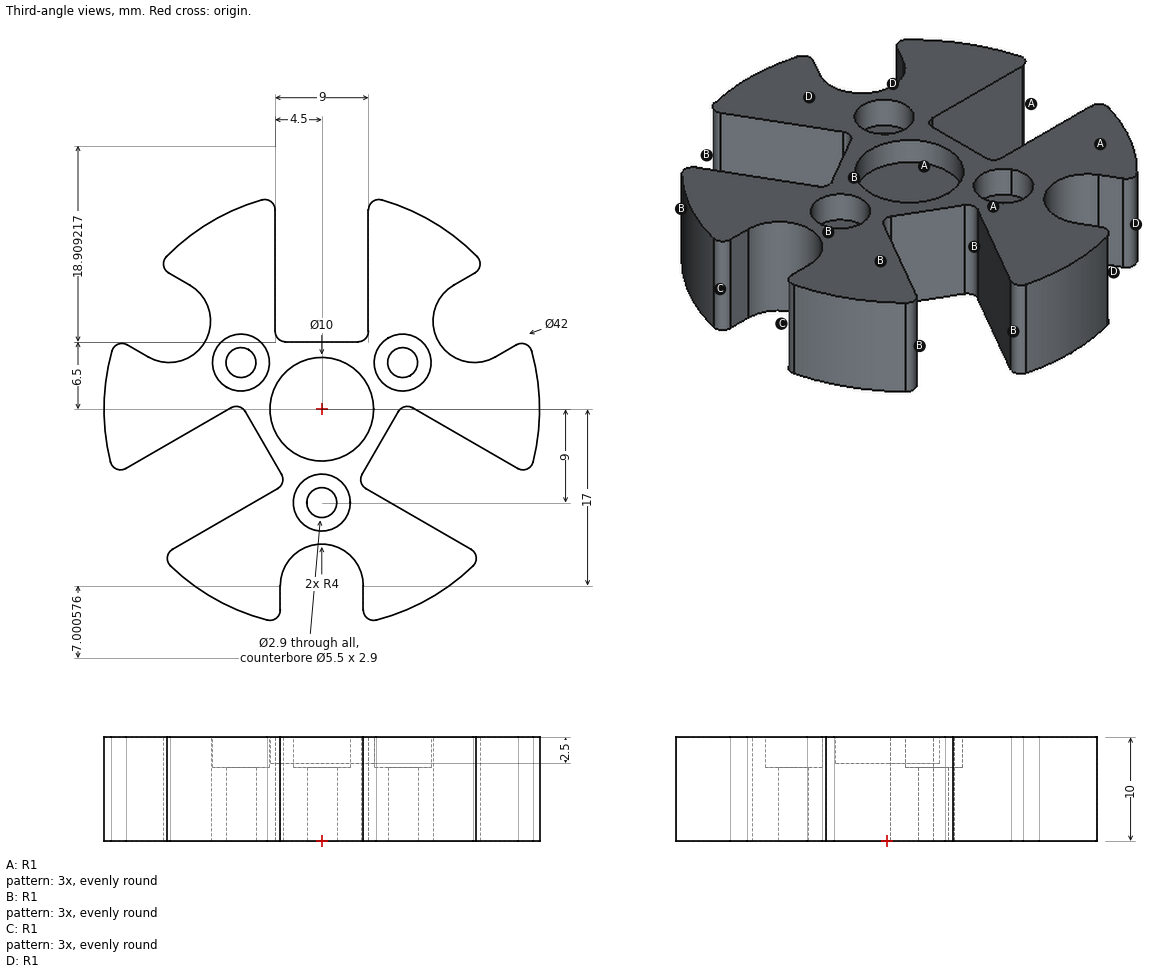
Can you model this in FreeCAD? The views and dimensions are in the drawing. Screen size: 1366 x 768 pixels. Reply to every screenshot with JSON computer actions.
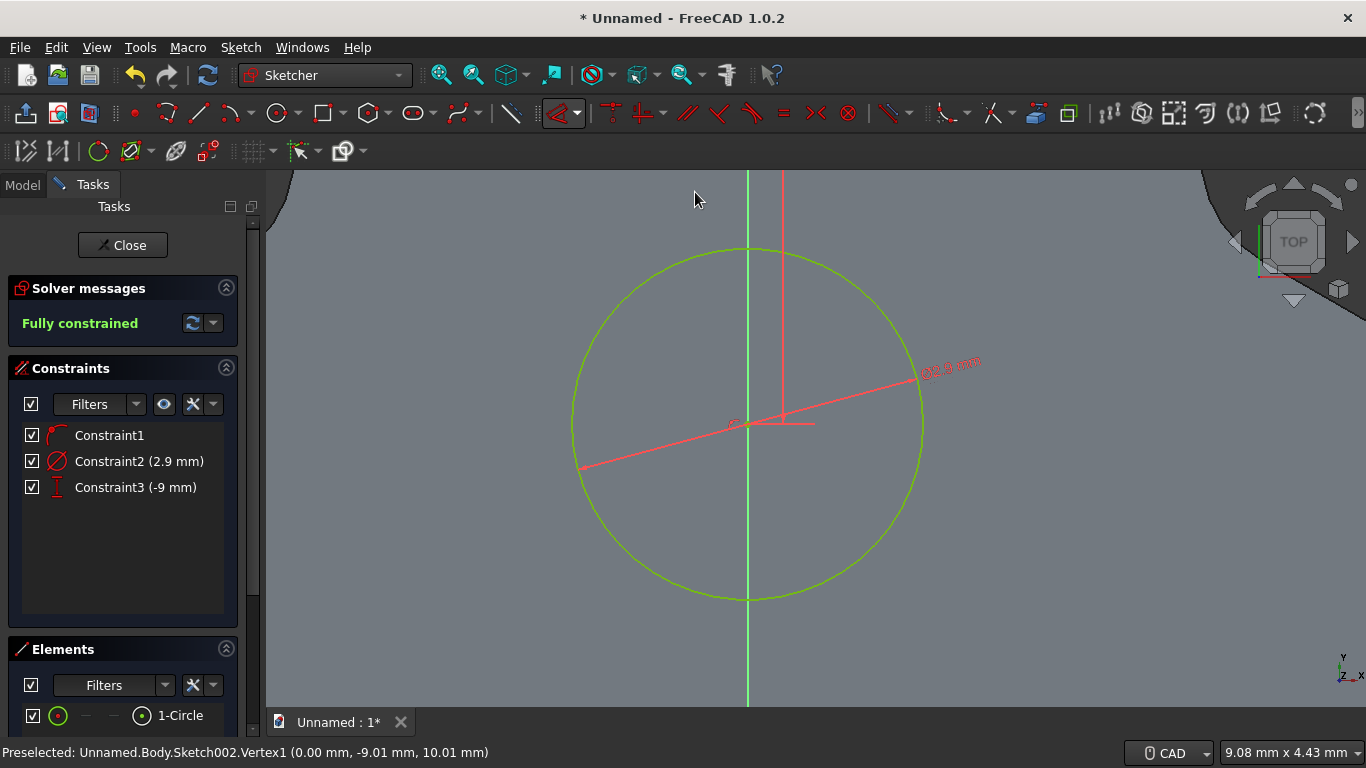
{"action": "left_click", "coordinate": [123, 245]}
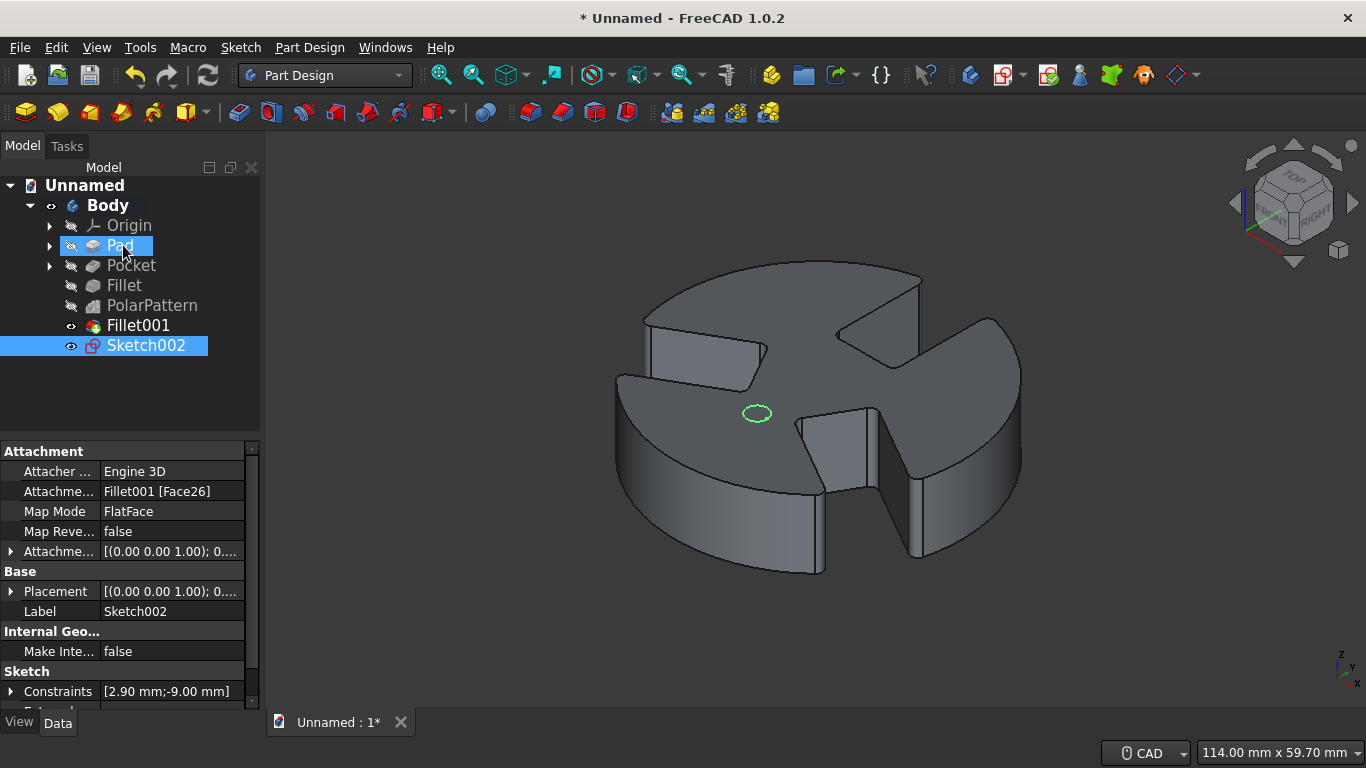
{"action": "left_click", "coordinate": [272, 112]}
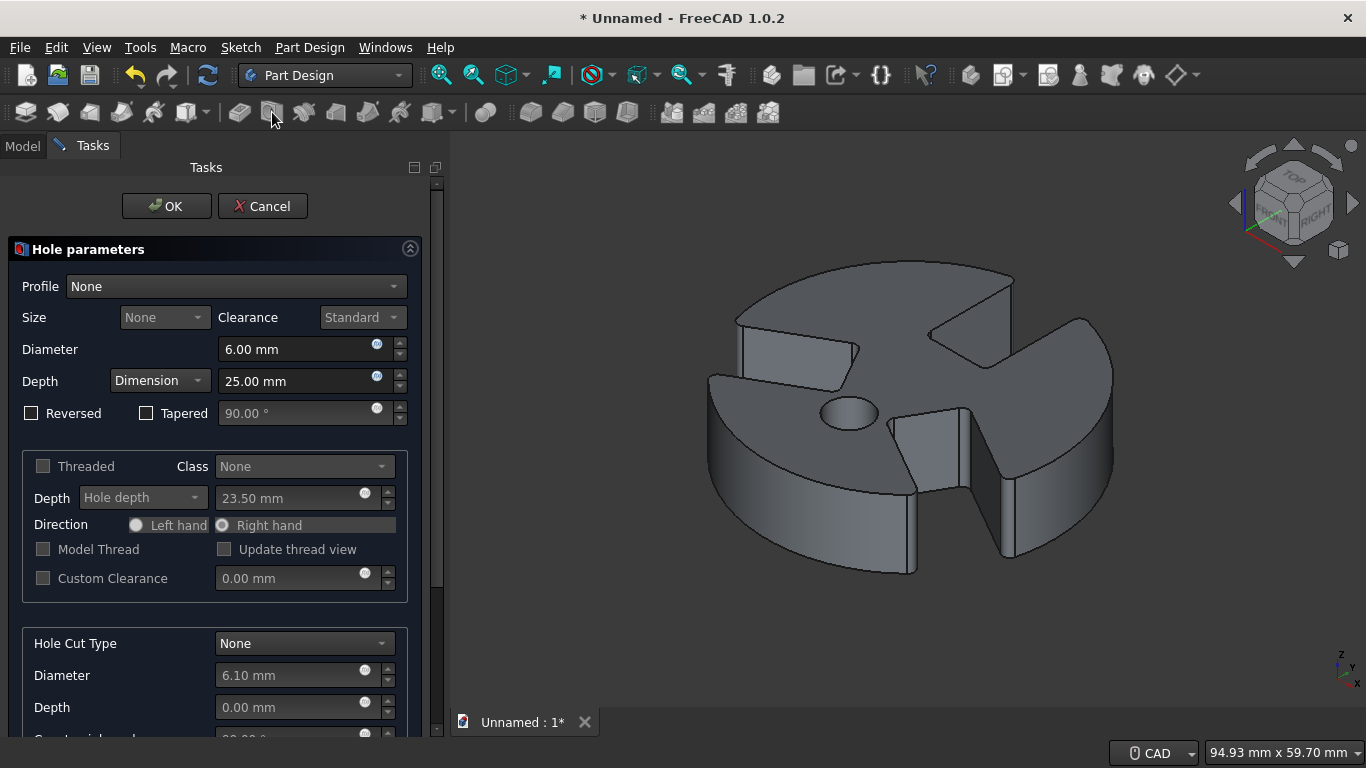
{"action": "triple_click", "coordinate": [305, 349]}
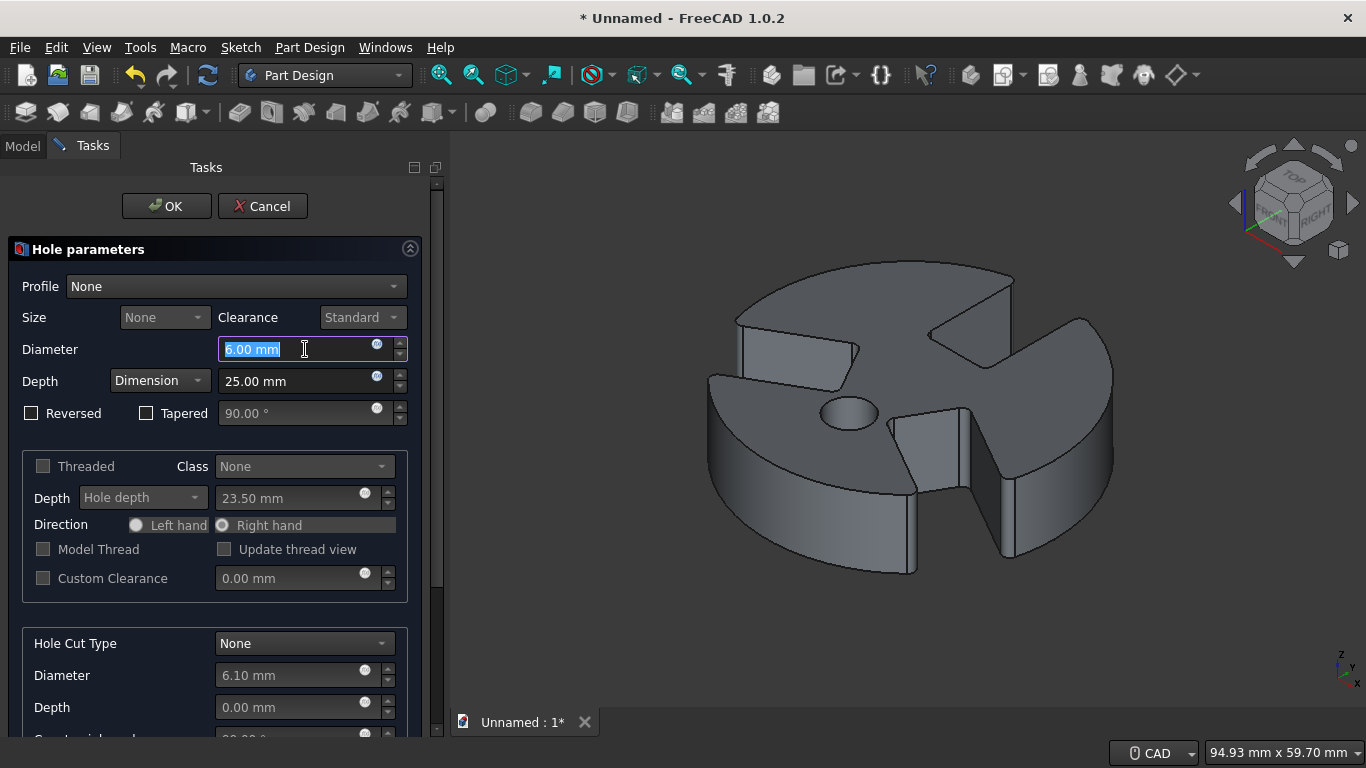
{"action": "type", "text": "2.9"}
{"action": "key", "text": "Tab"}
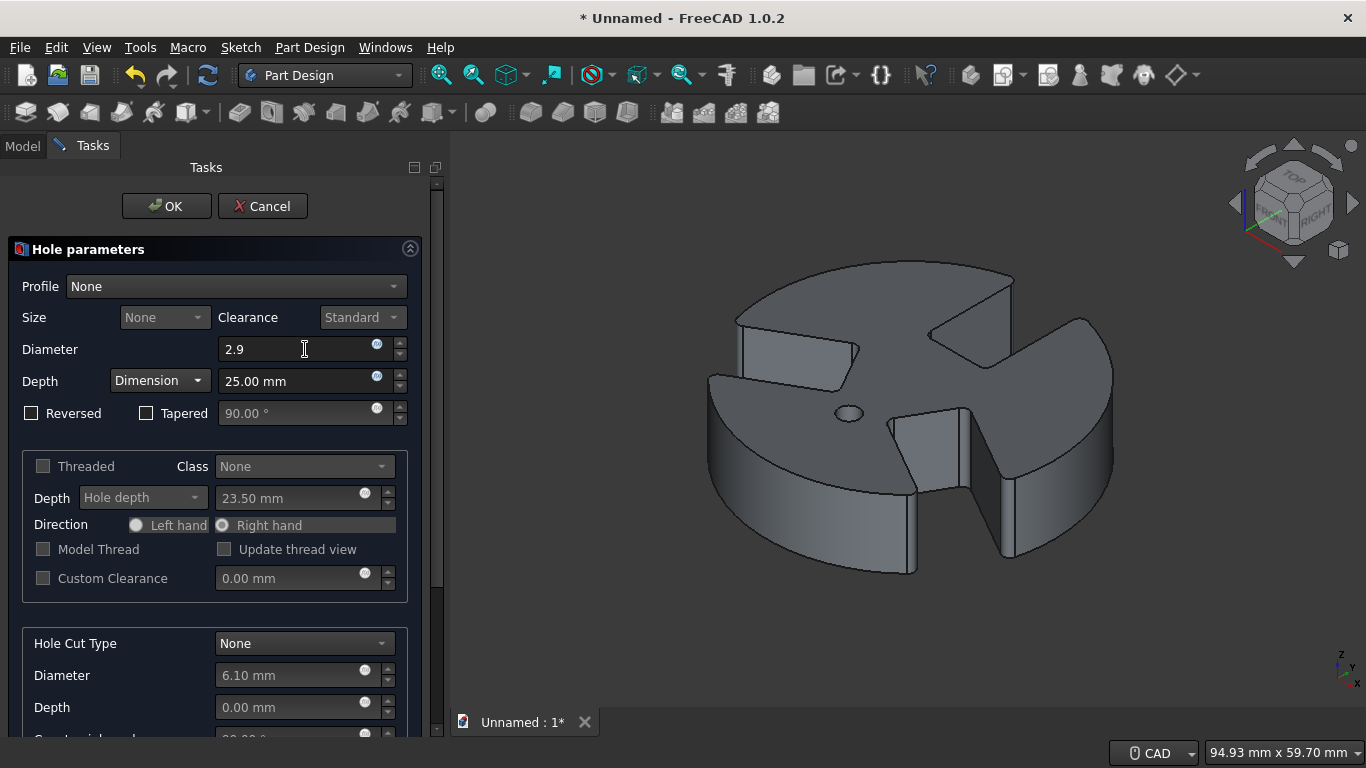
{"action": "left_click", "coordinate": [161, 380]}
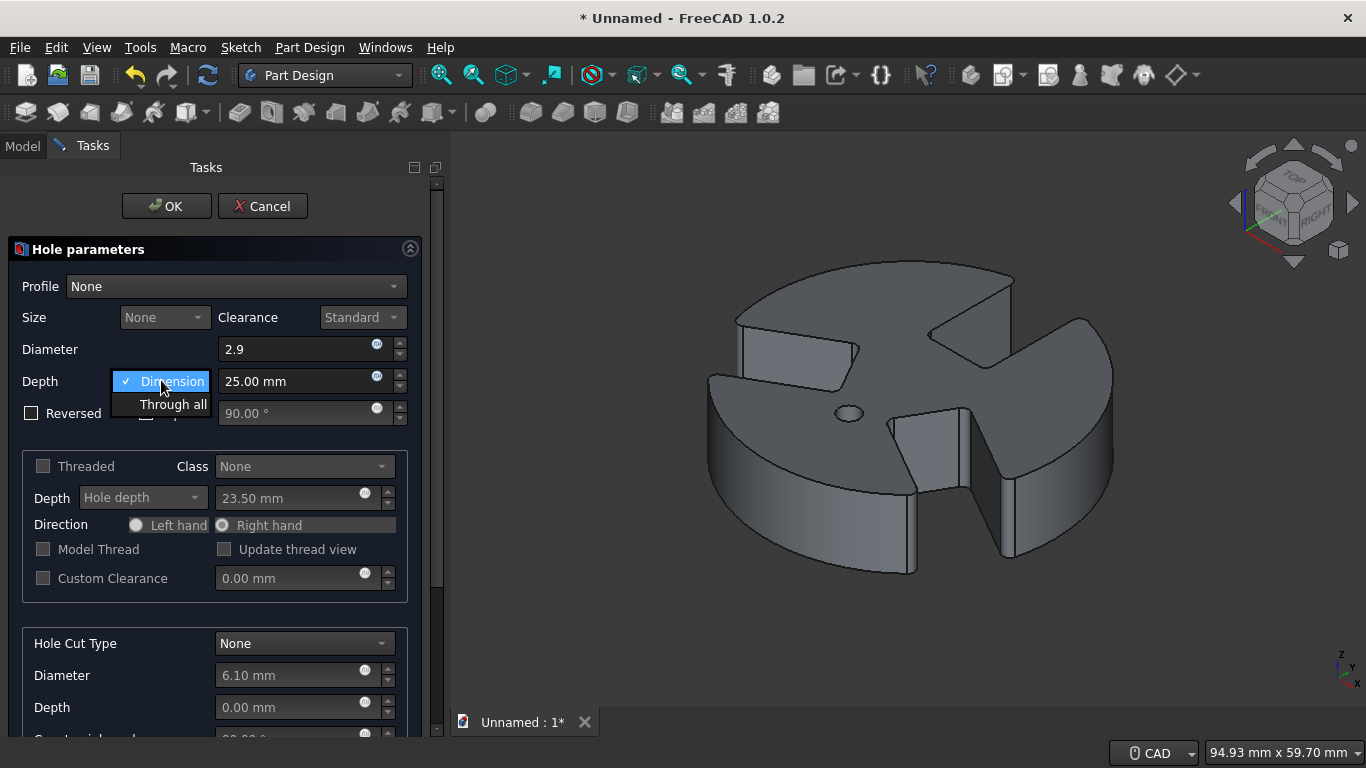
{"action": "left_click", "coordinate": [160, 404]}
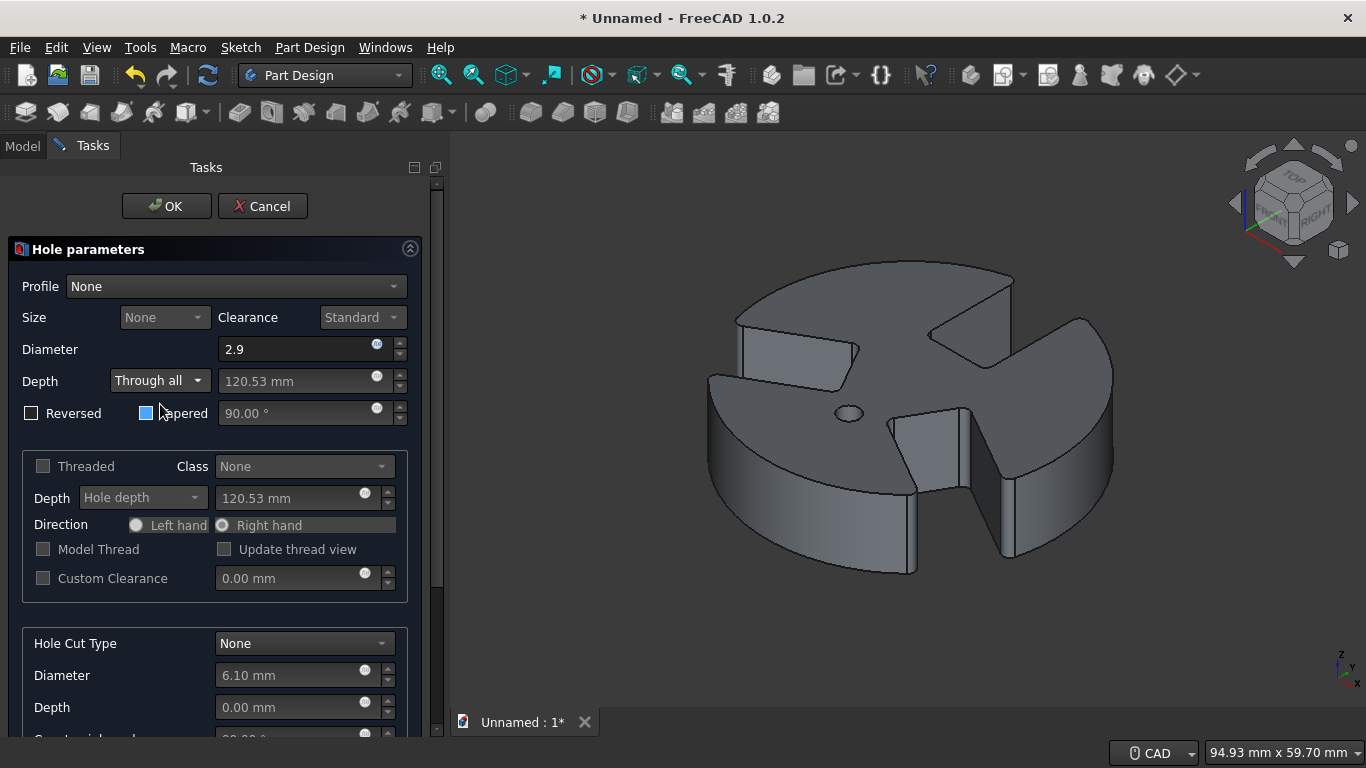
{"action": "left_click", "coordinate": [306, 644]}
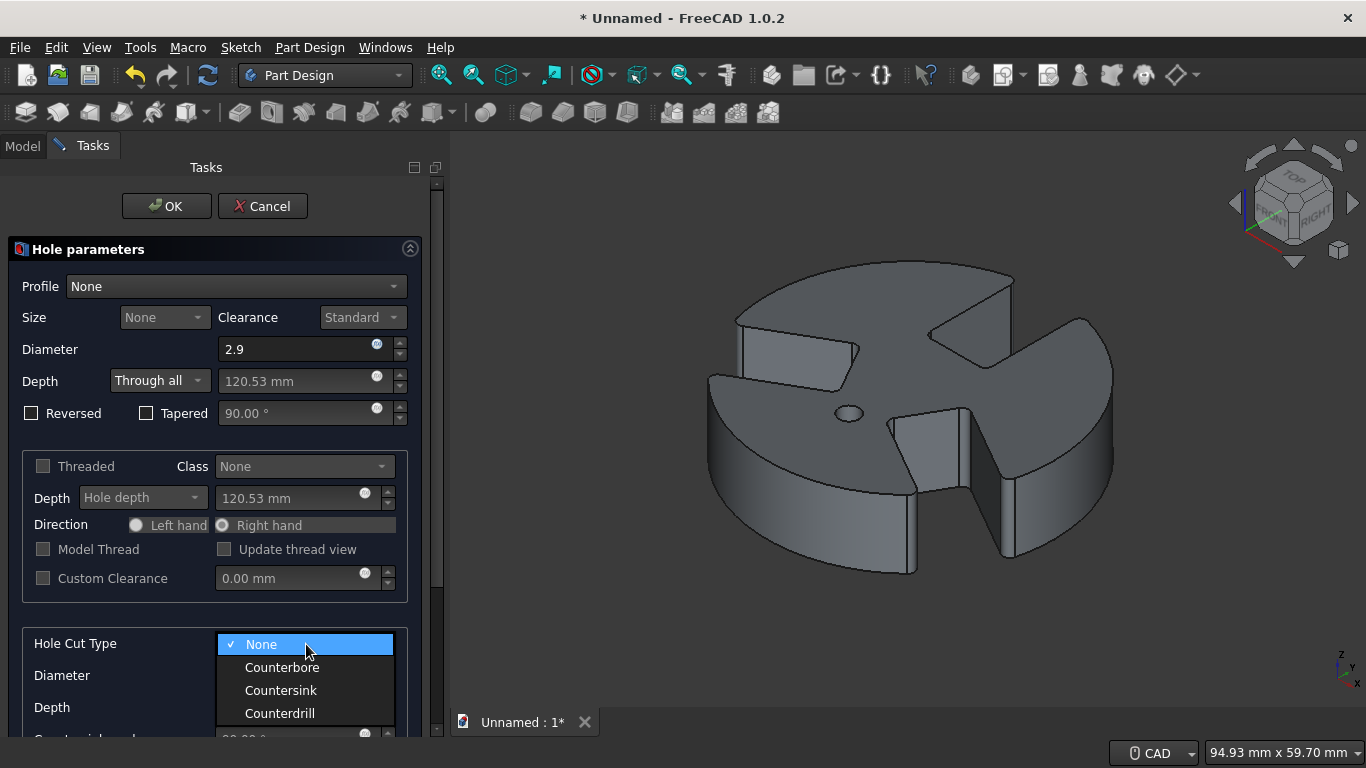
{"action": "left_click", "coordinate": [304, 668]}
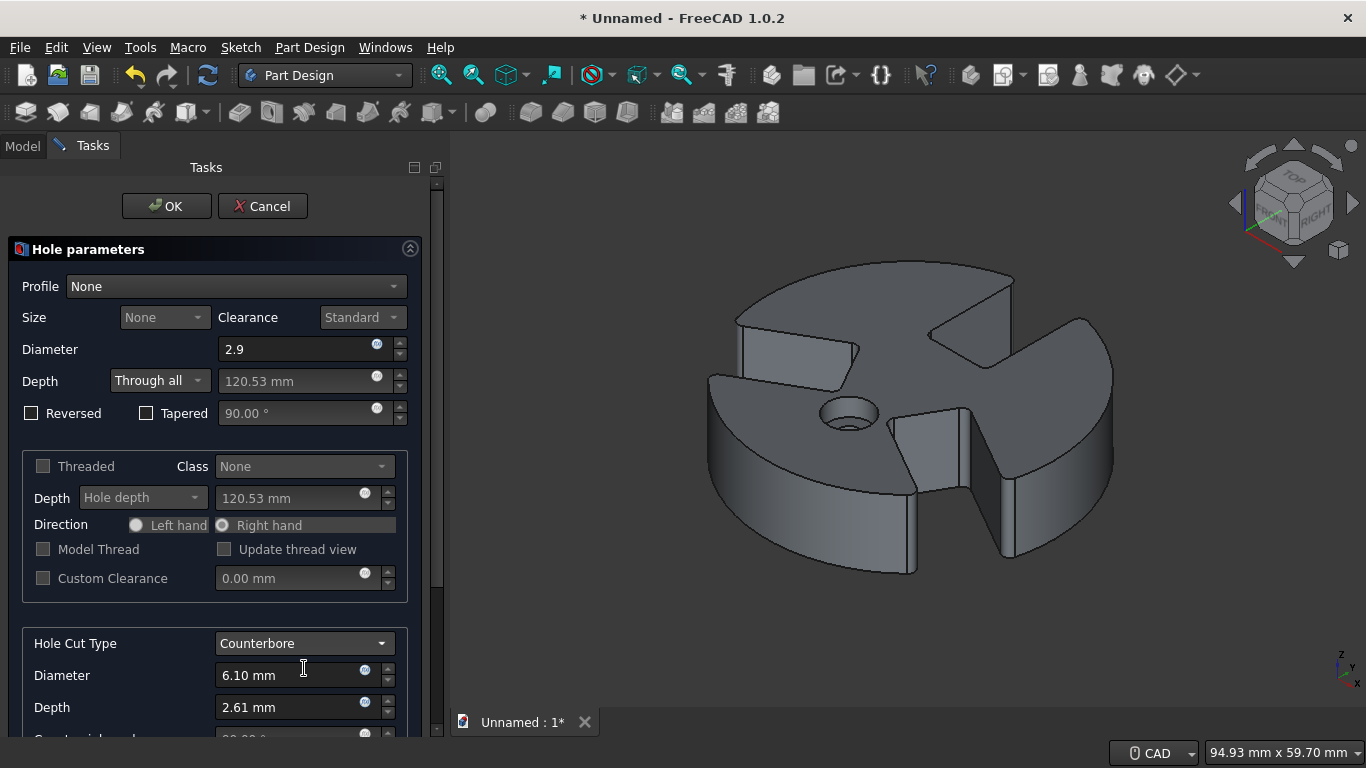
{"action": "triple_click", "coordinate": [298, 675]}